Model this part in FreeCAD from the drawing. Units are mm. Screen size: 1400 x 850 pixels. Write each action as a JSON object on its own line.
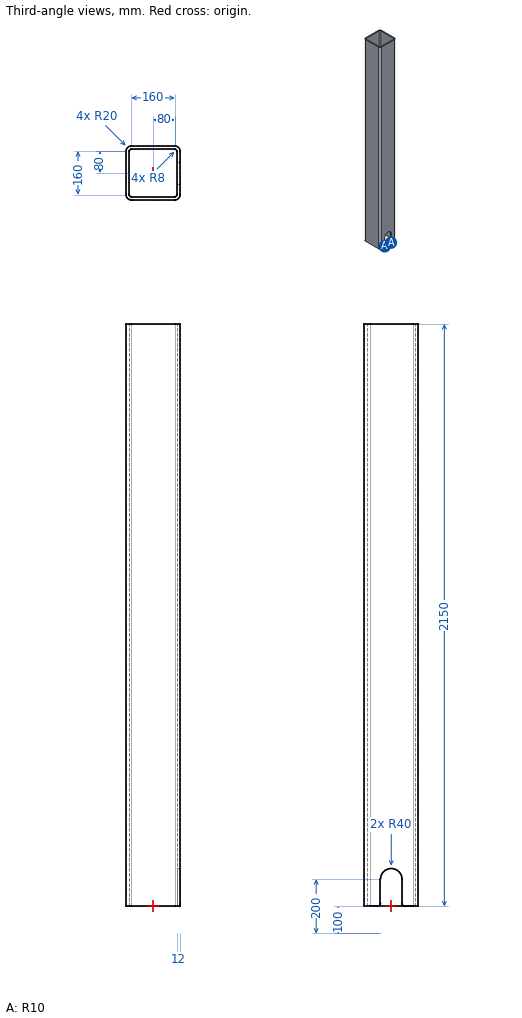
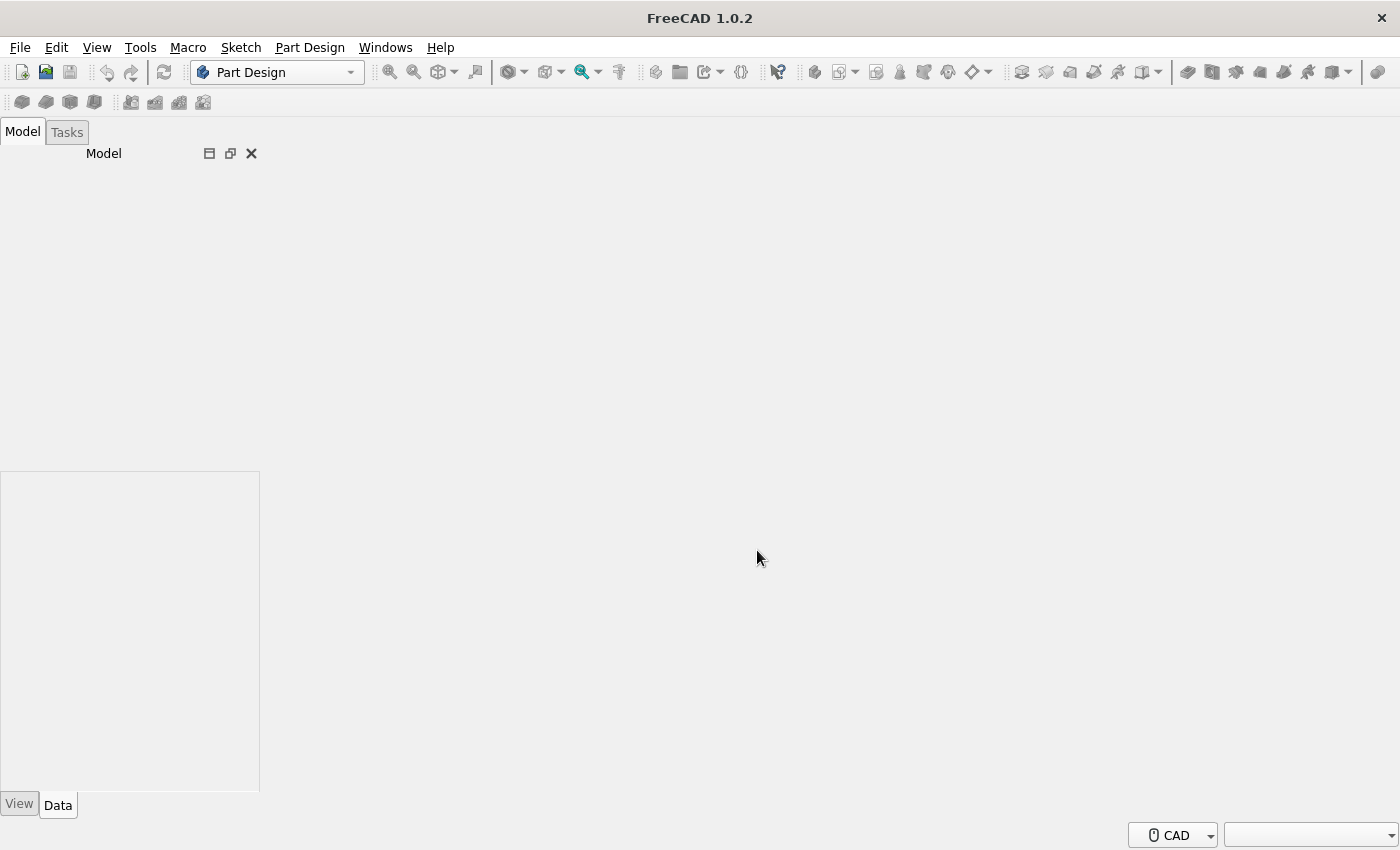
{"action": "left_click", "coordinate": [22, 72]}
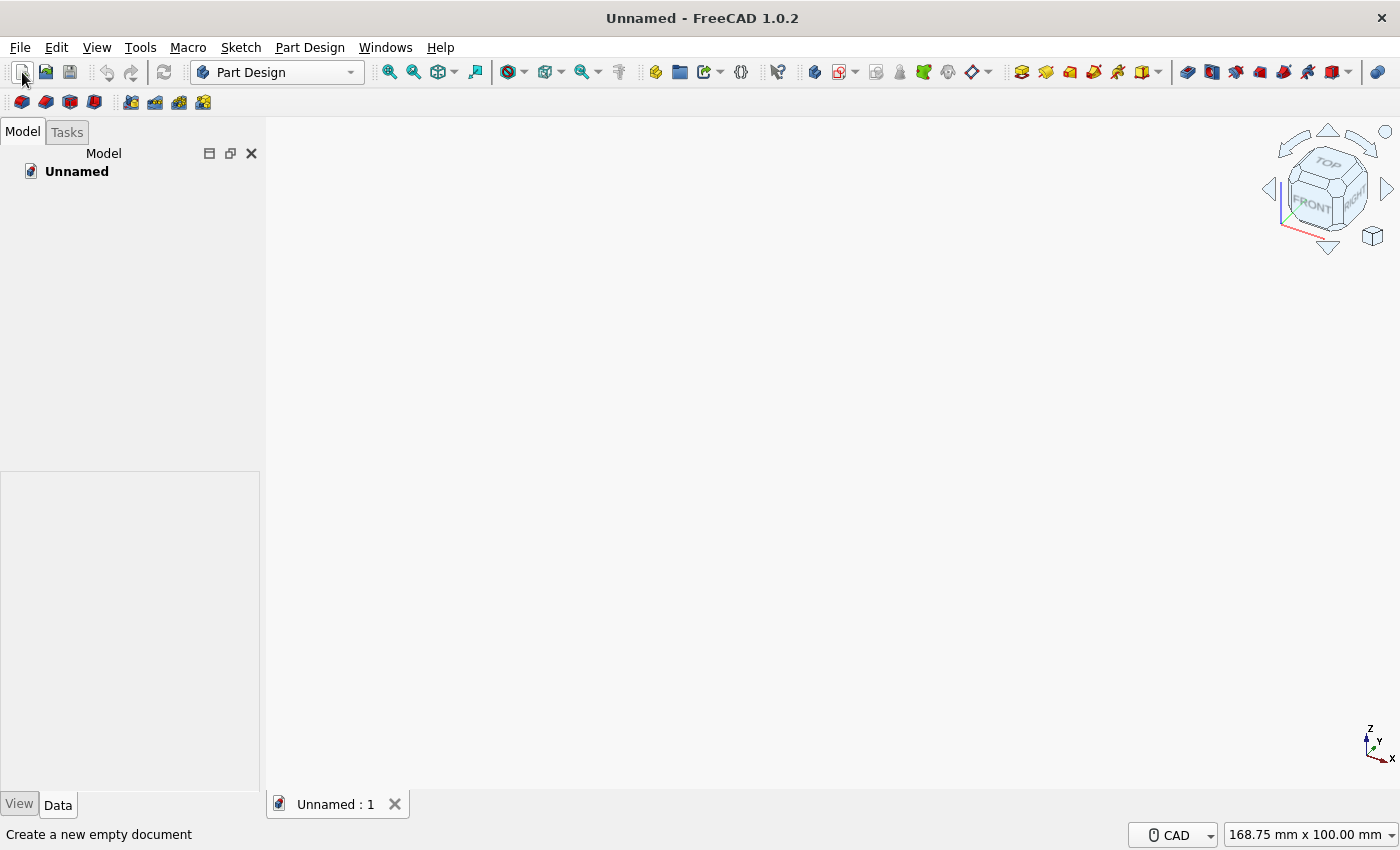
{"action": "left_click", "coordinate": [840, 72]}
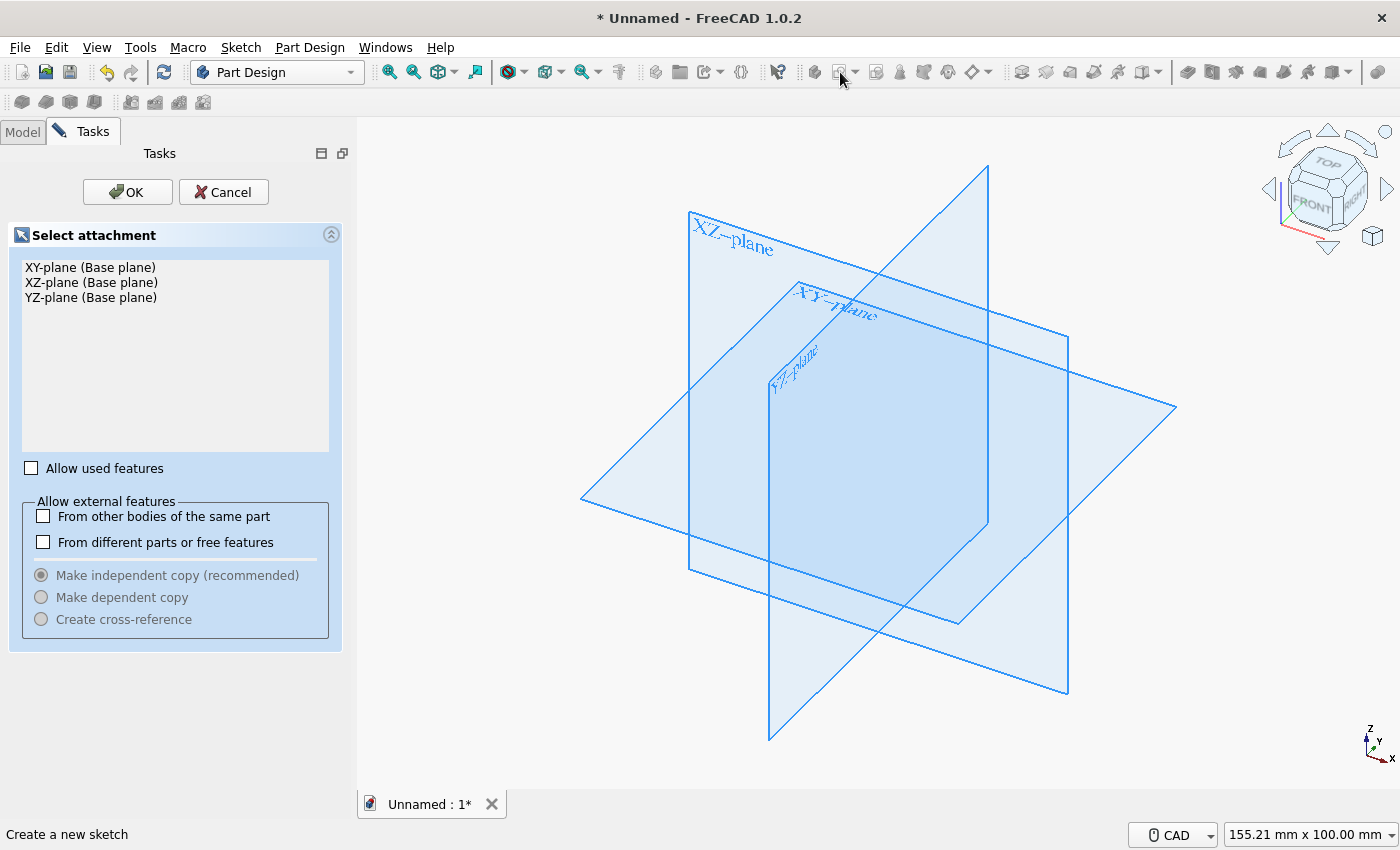
{"action": "left_click", "coordinate": [82, 268]}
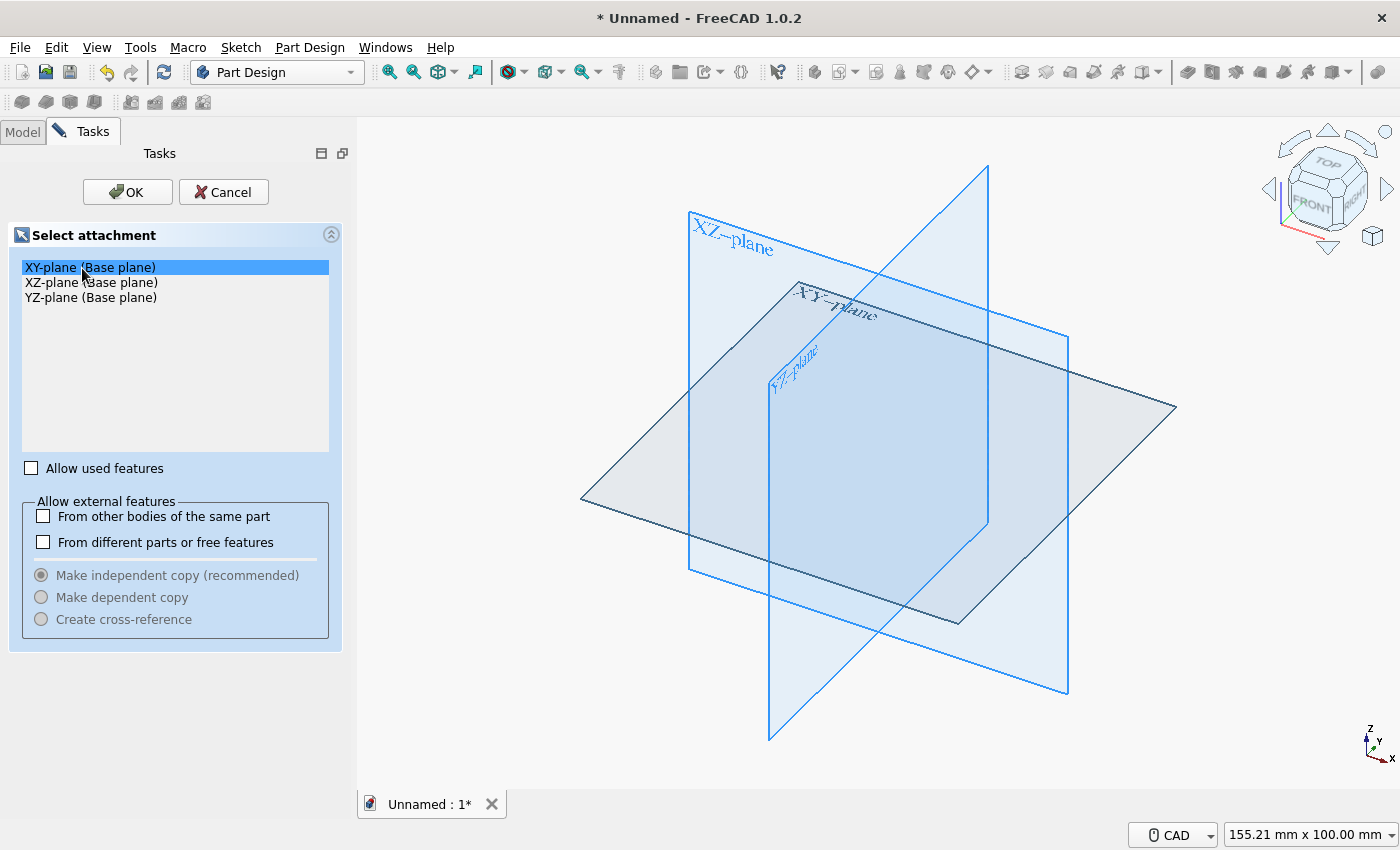
{"action": "left_click", "coordinate": [128, 192]}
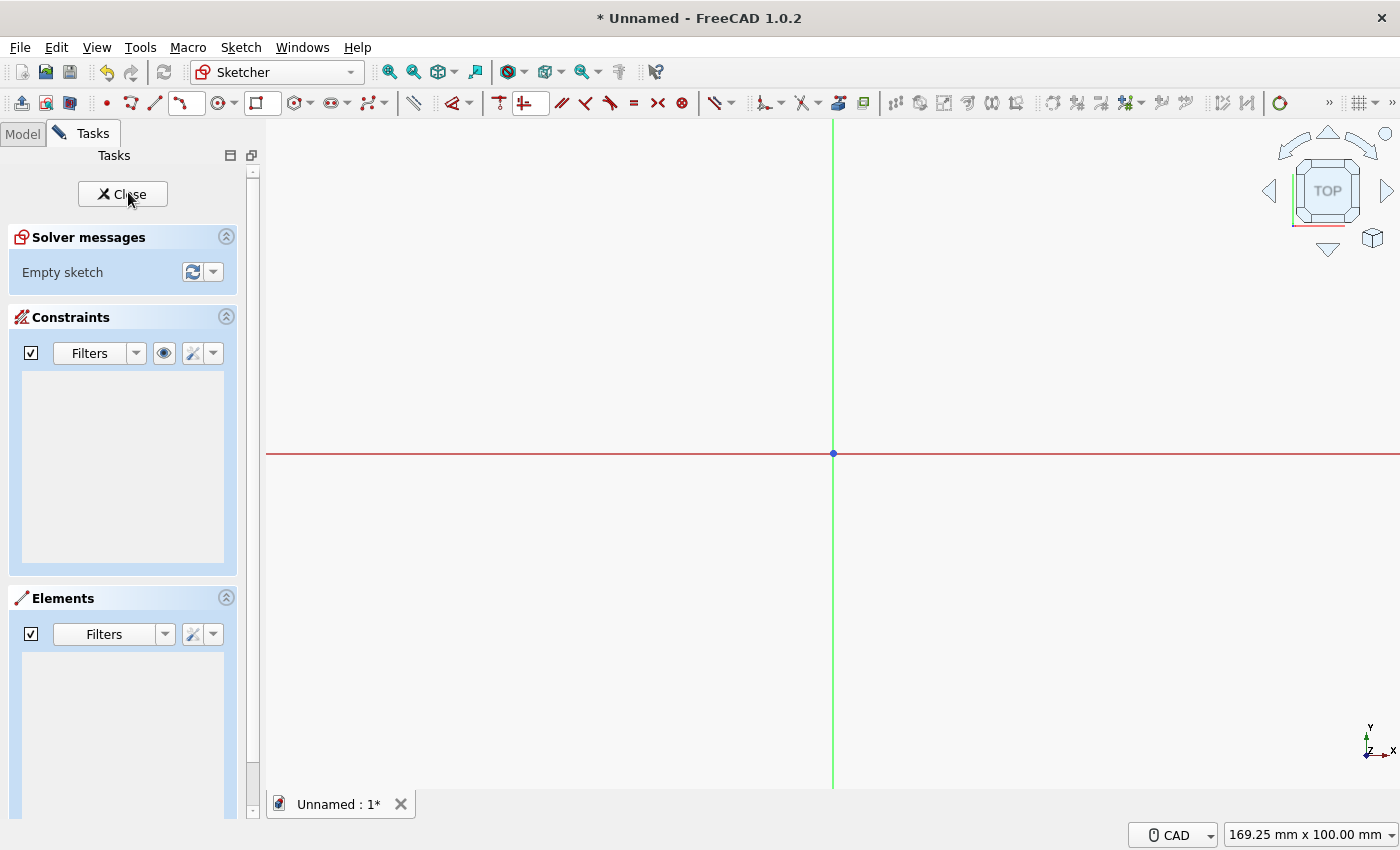
{"action": "scroll", "coordinate": [735, 454], "scroll_direction": "down", "scroll_amount": 6}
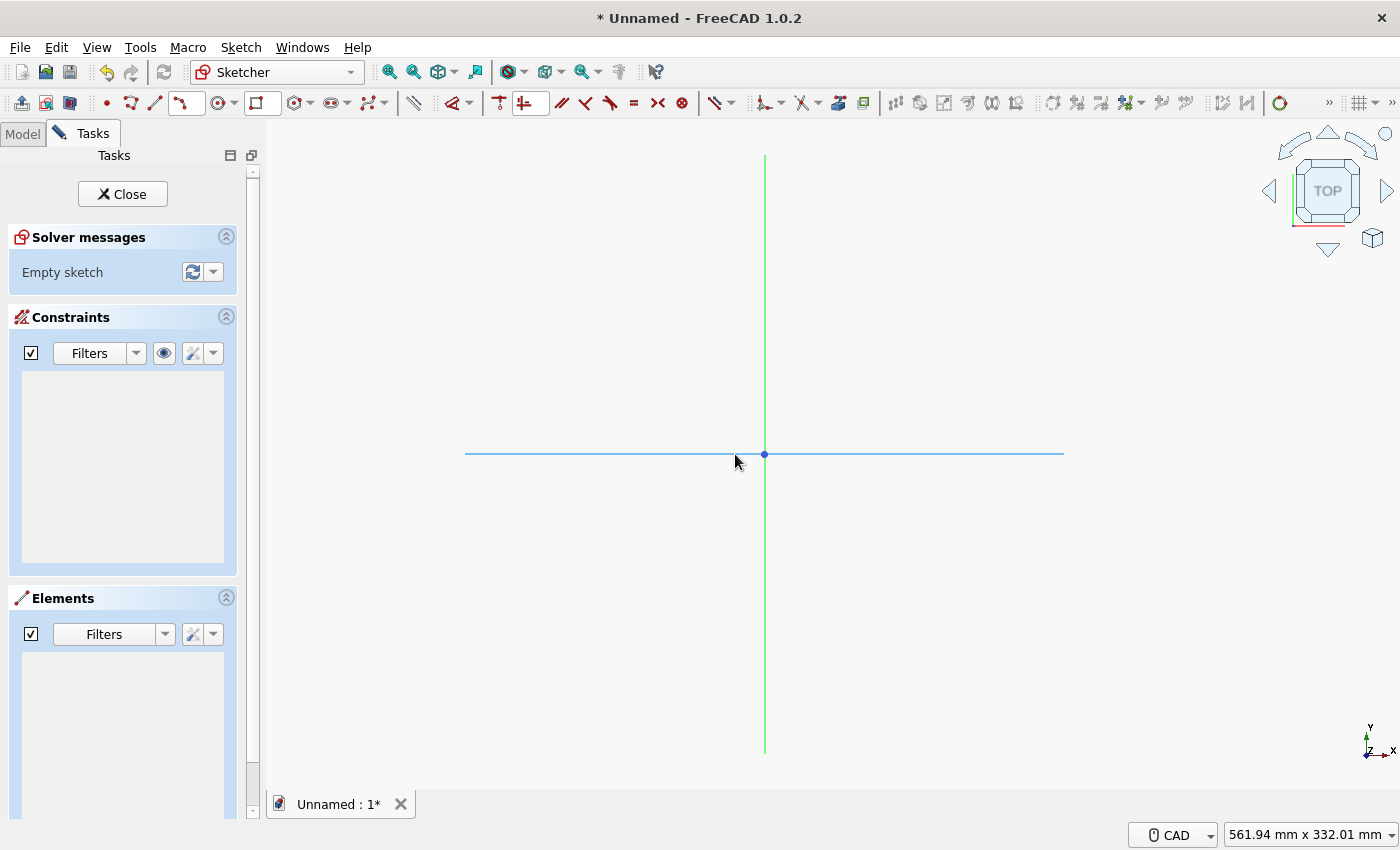
{"action": "left_click", "coordinate": [156, 104]}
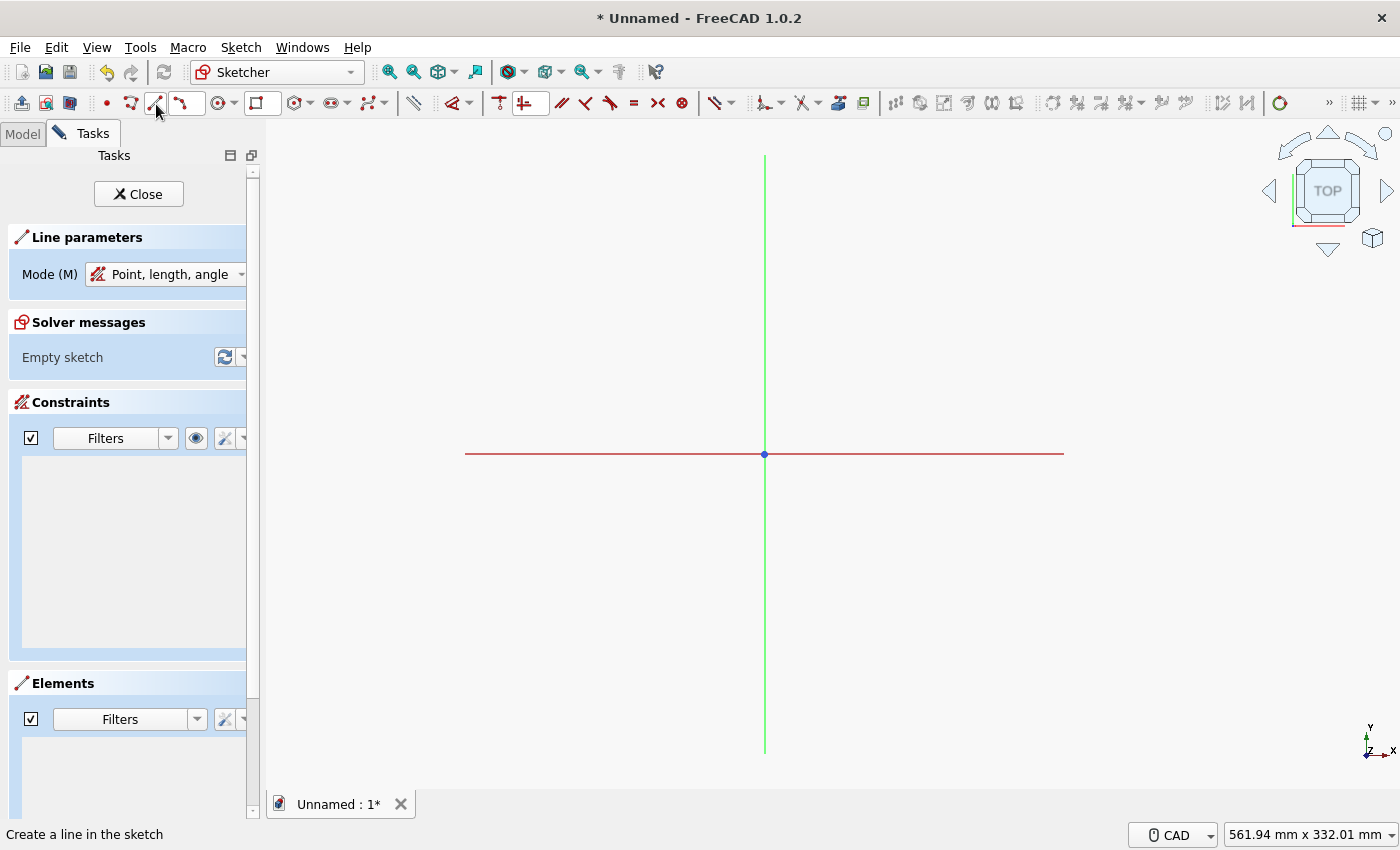
{"action": "left_click", "coordinate": [926, 253]}
{"action": "left_click", "coordinate": [603, 253]}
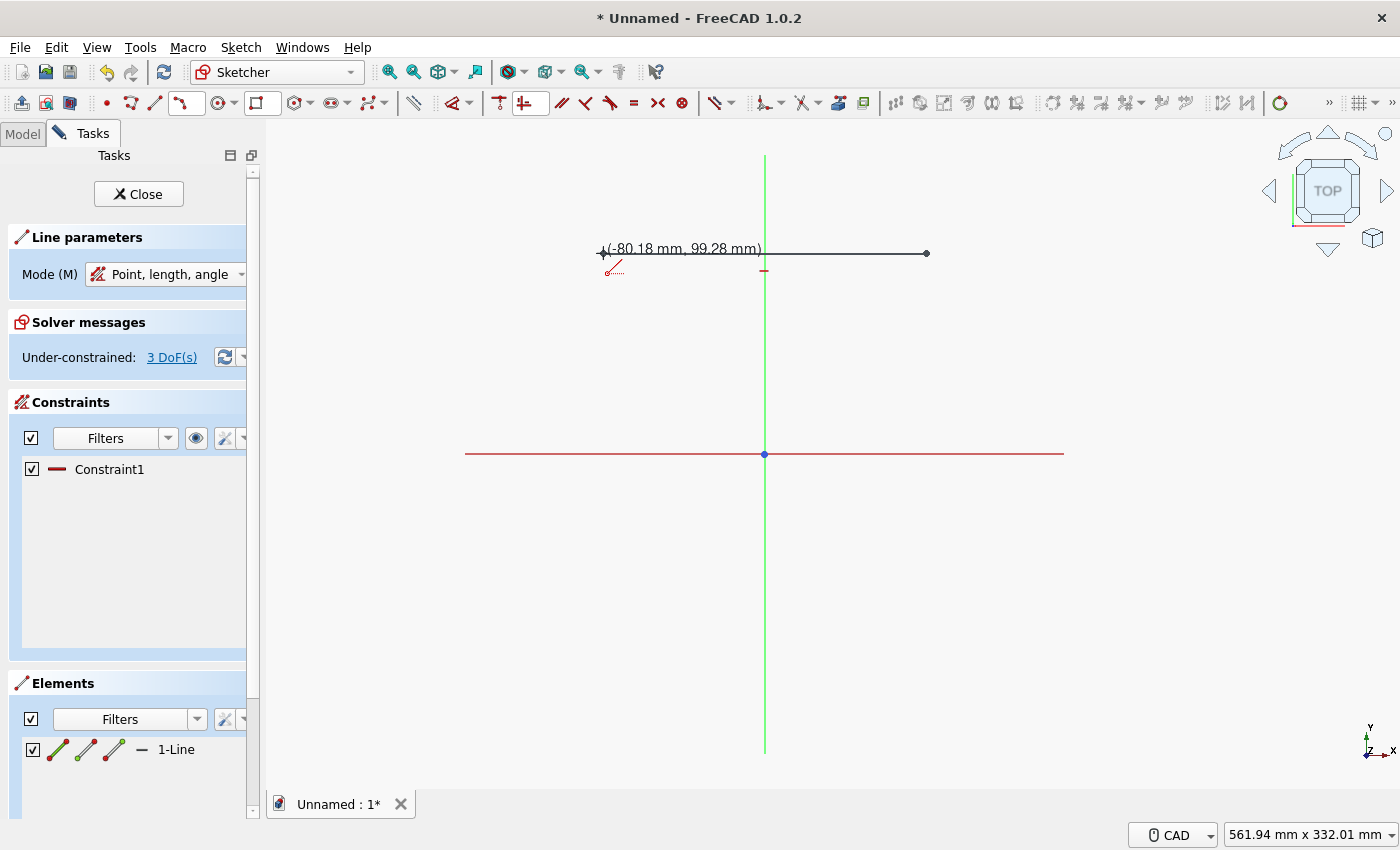
{"action": "left_click", "coordinate": [563, 293]}
{"action": "left_click", "coordinate": [563, 616]}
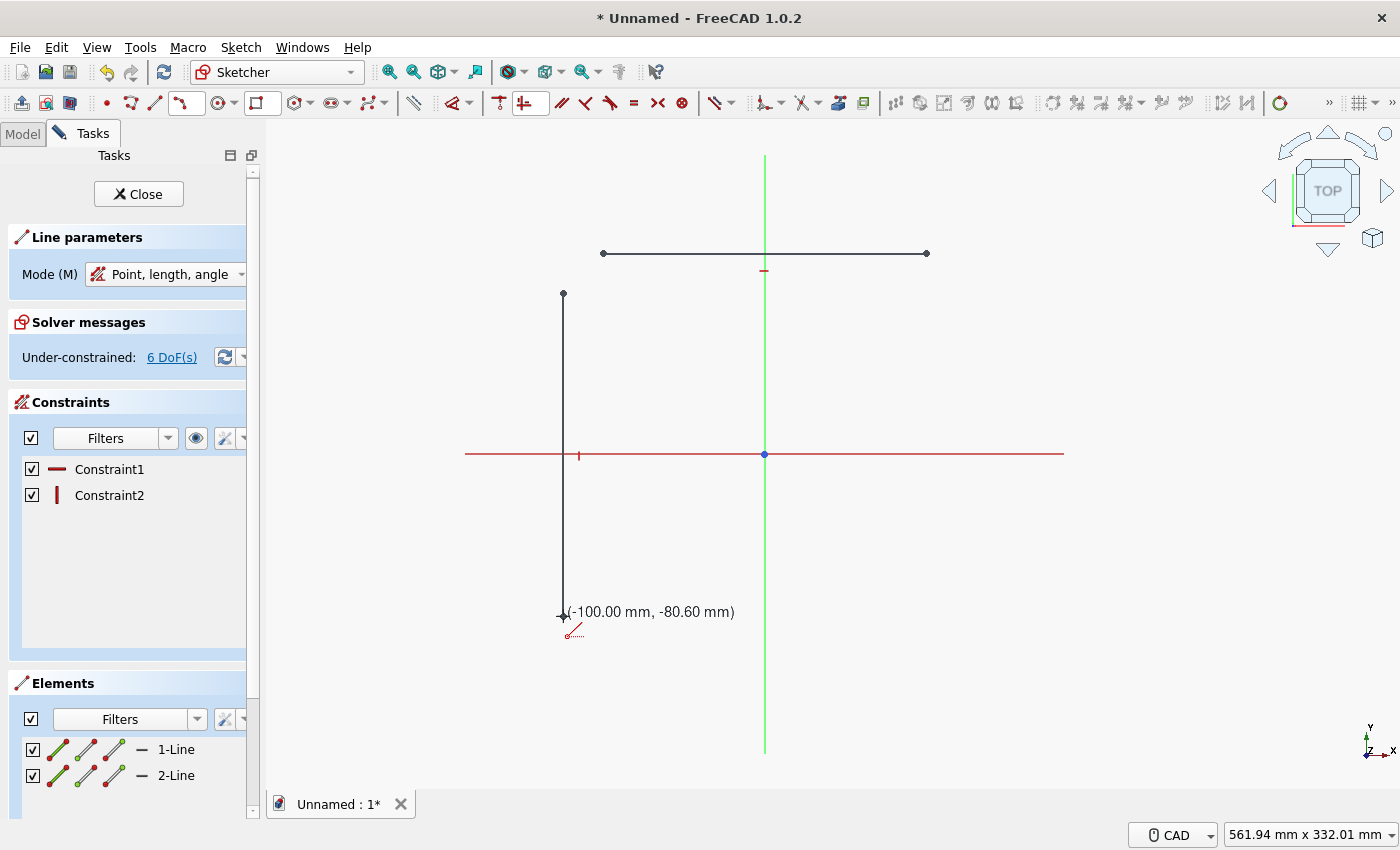
{"action": "left_click", "coordinate": [603, 656]}
{"action": "left_click", "coordinate": [926, 656]}